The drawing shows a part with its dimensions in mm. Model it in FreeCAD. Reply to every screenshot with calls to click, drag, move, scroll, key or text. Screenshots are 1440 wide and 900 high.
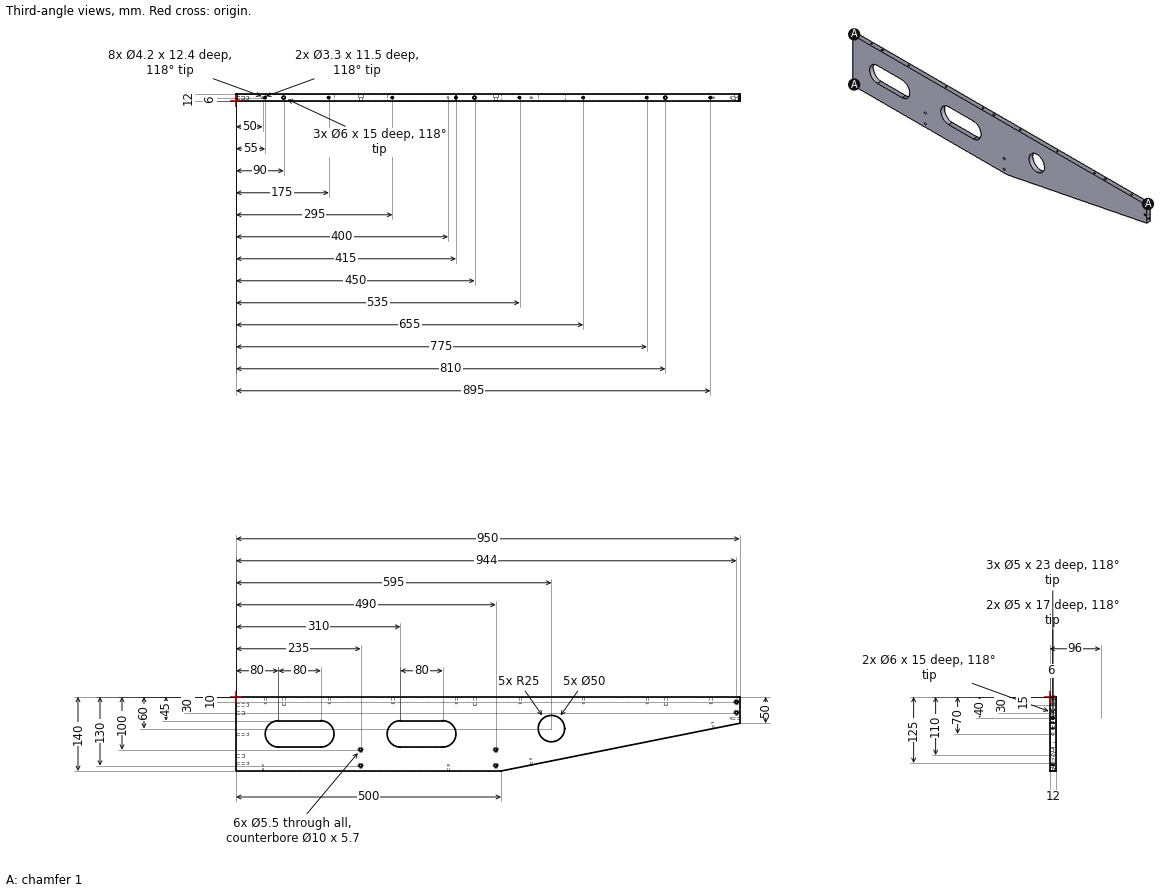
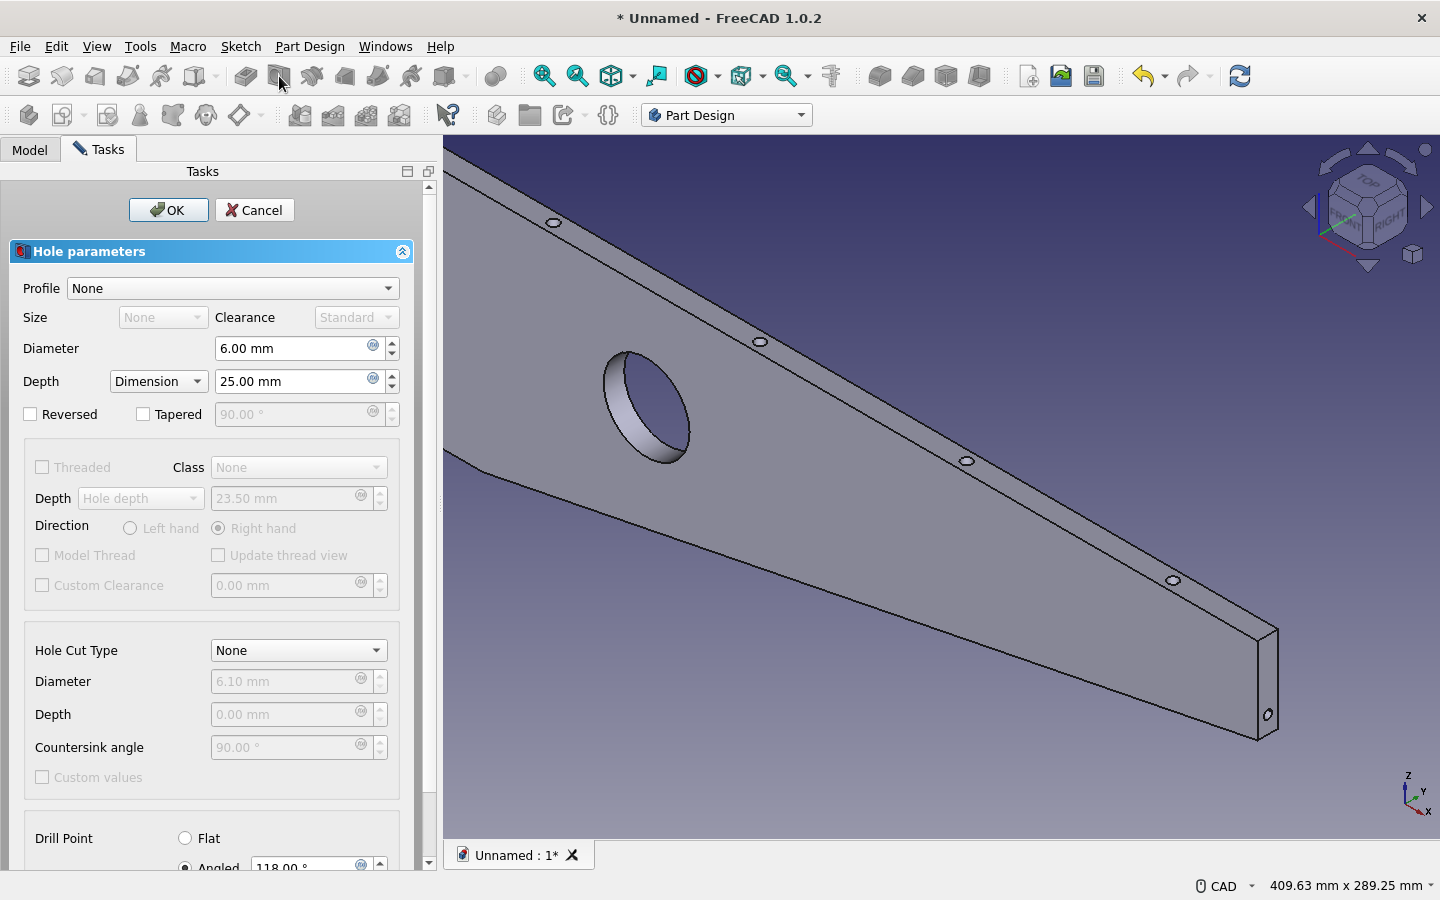
triple_click(300, 348)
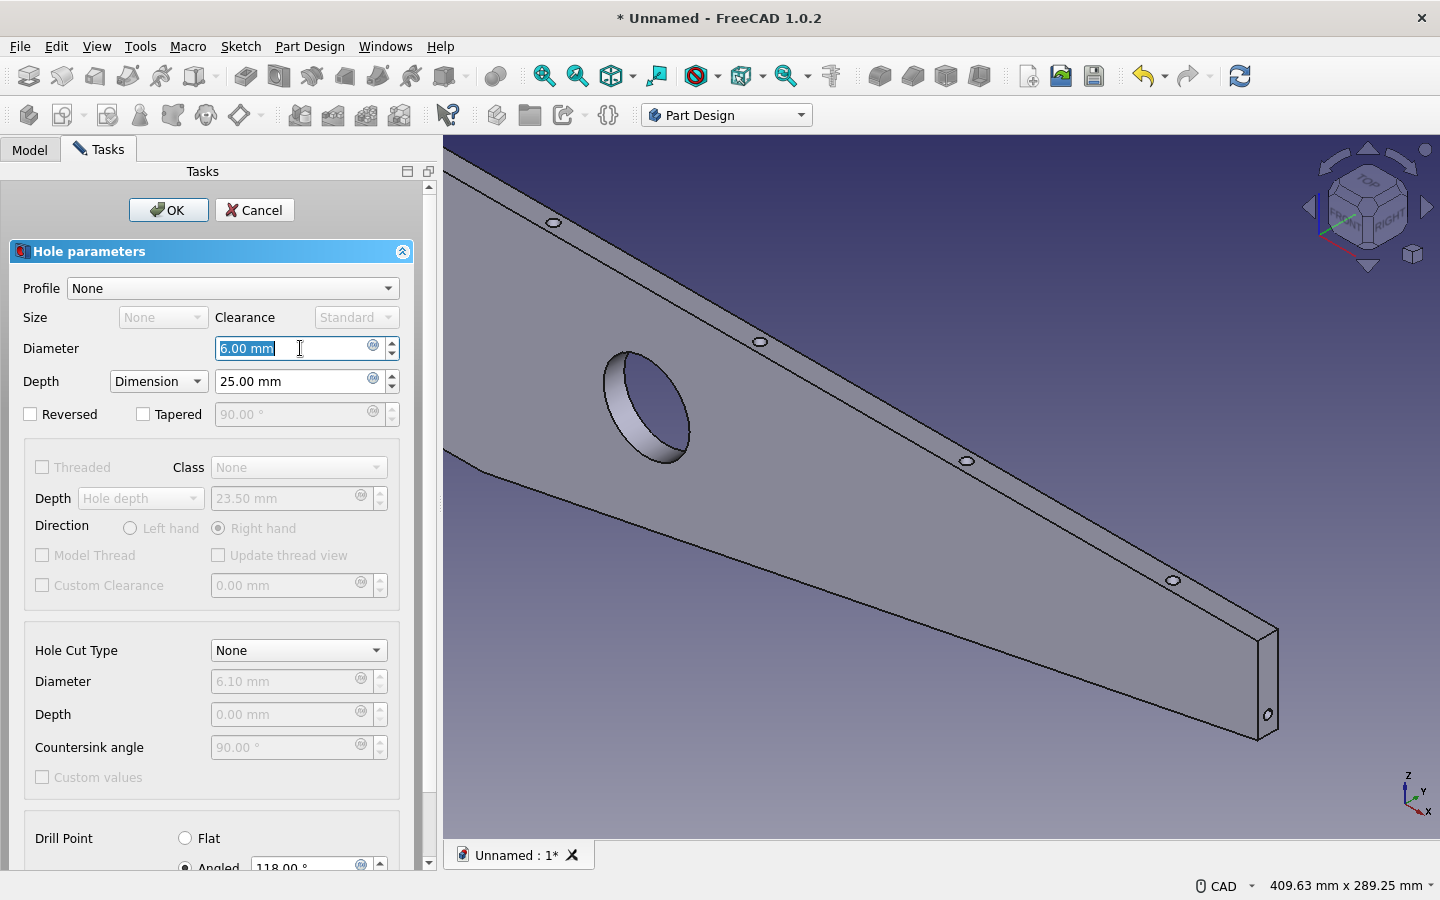
text(4.2)
key(Tab)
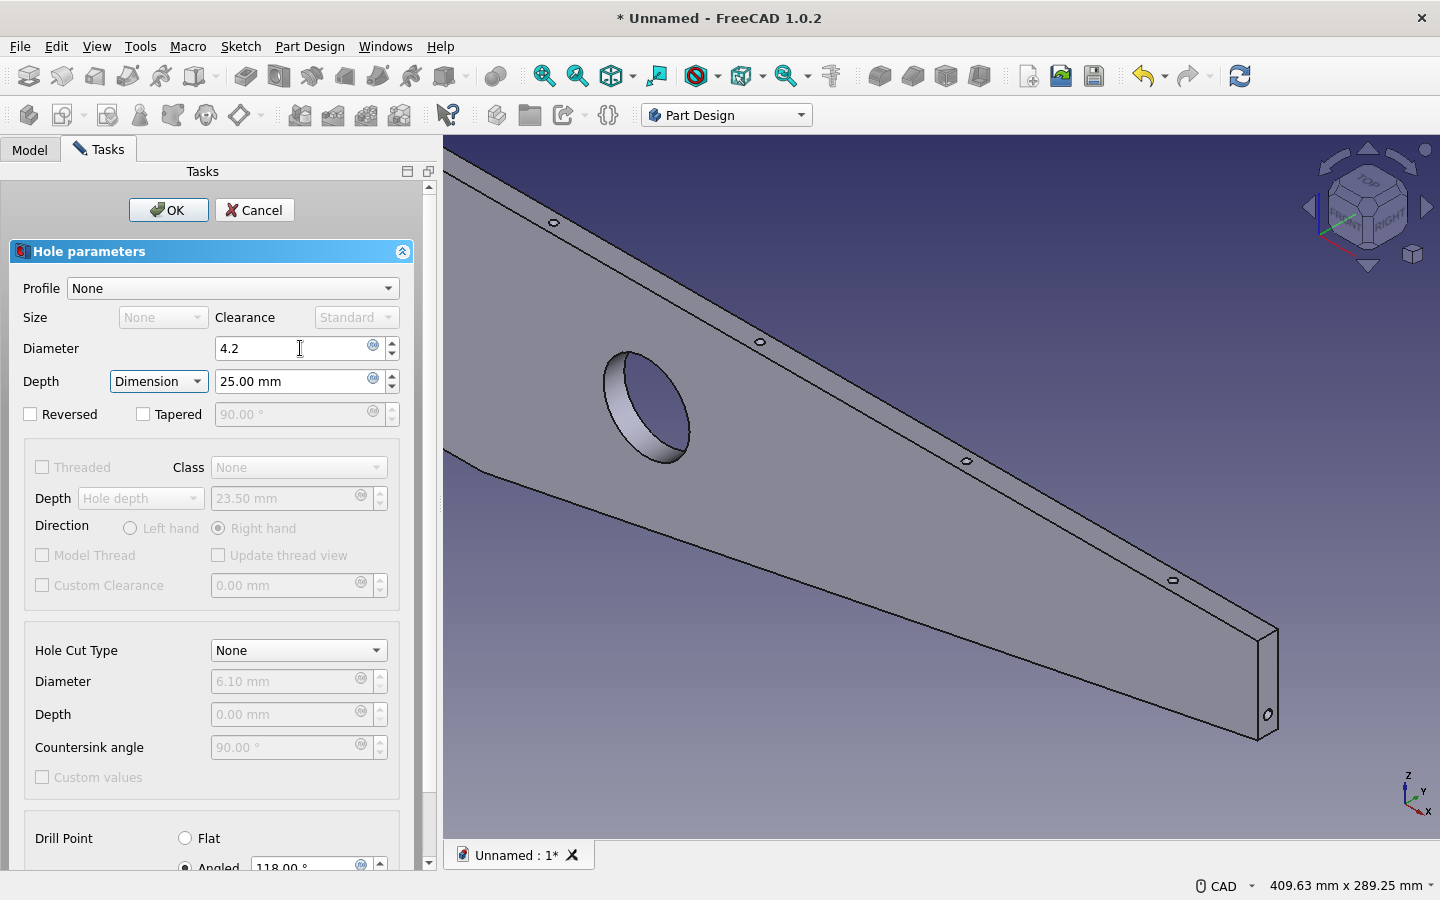
triple_click(300, 382)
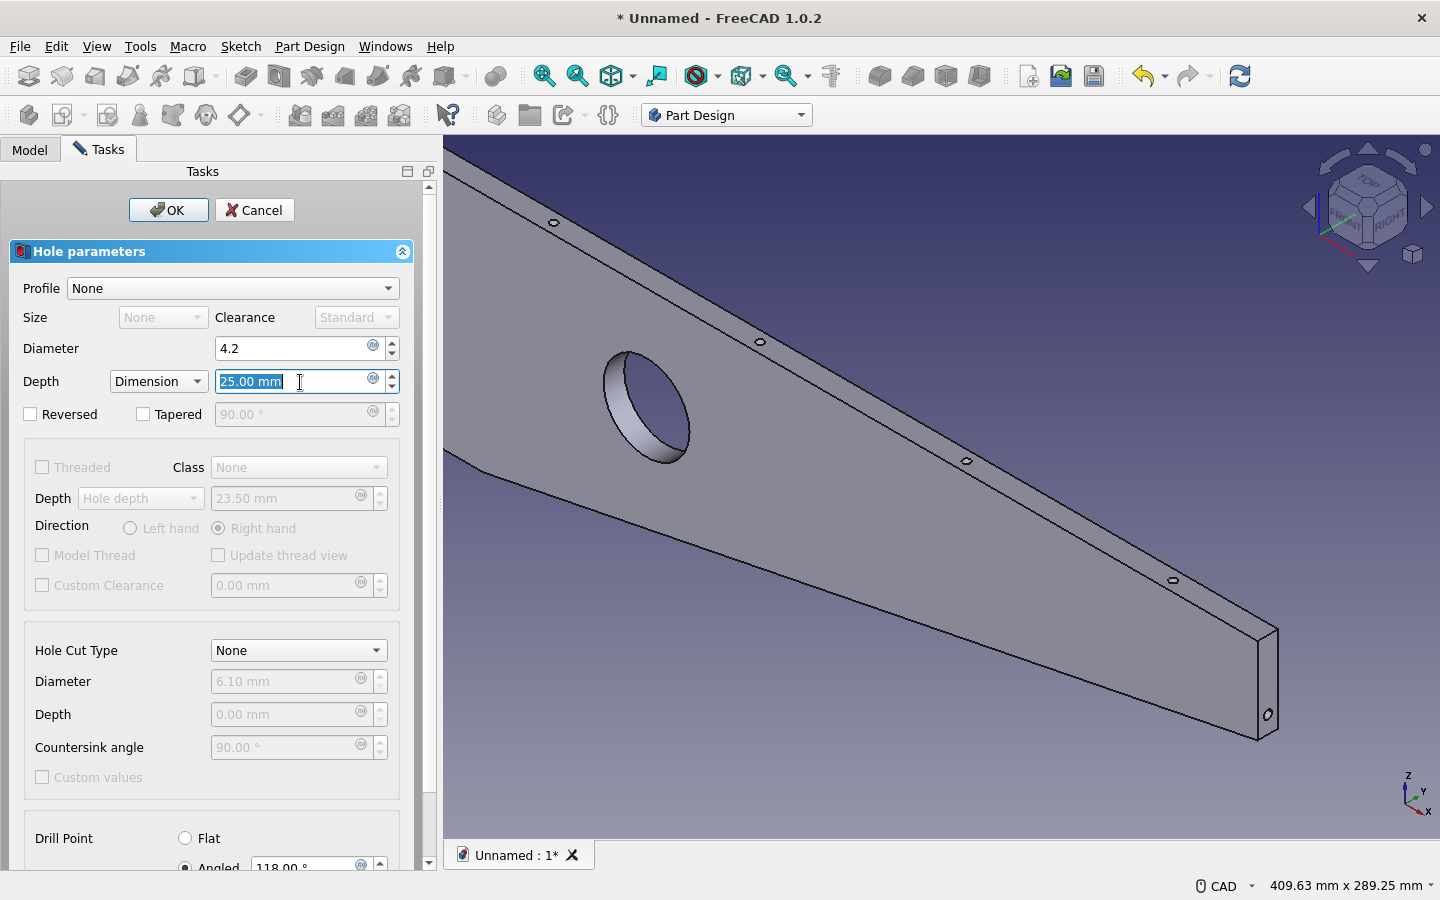
text(12.4)
key(Tab)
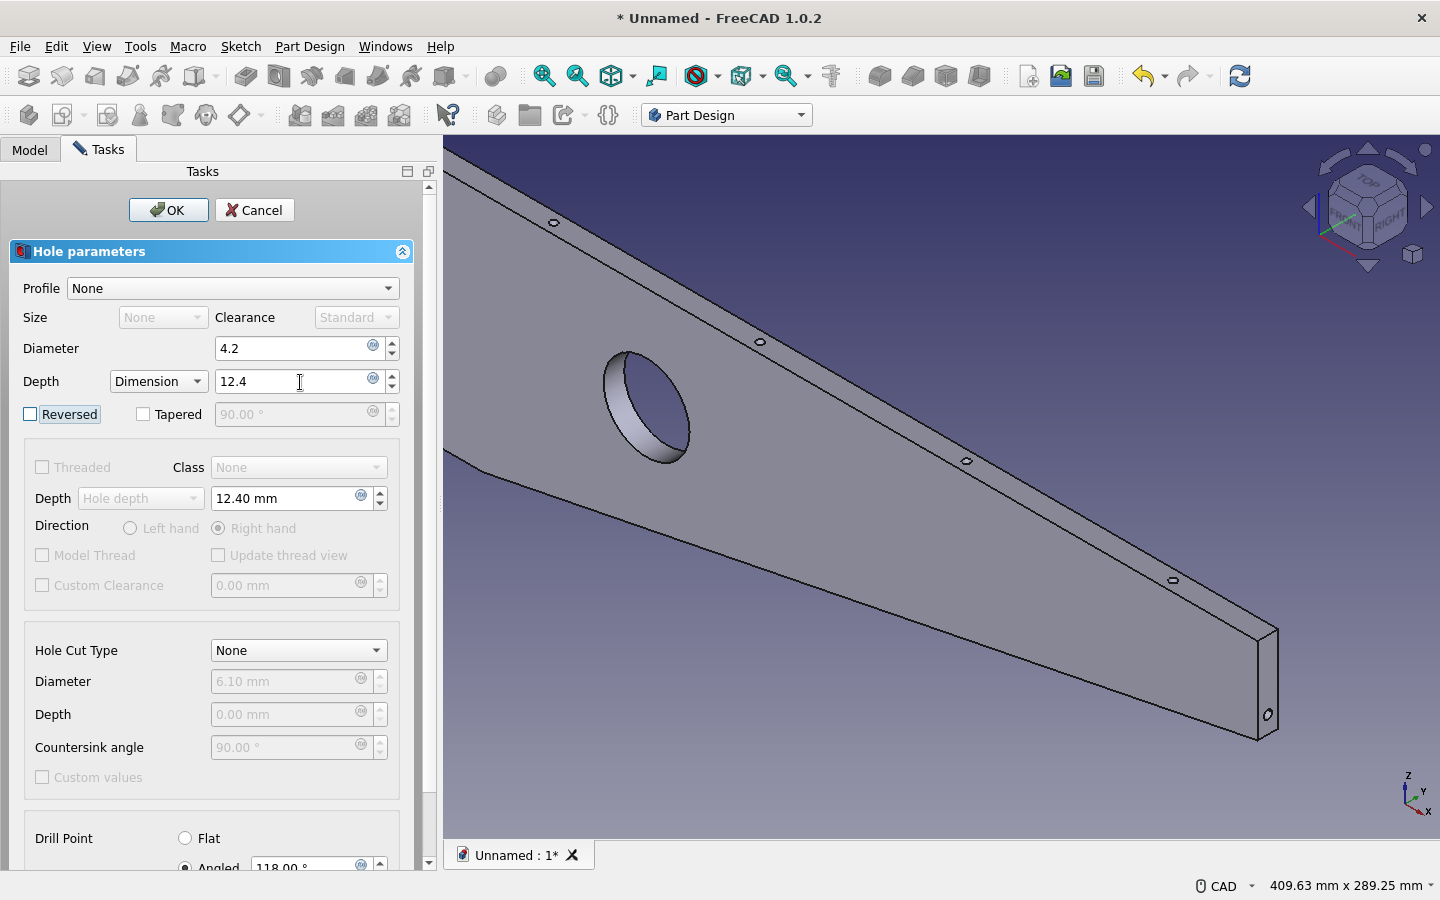
click(169, 210)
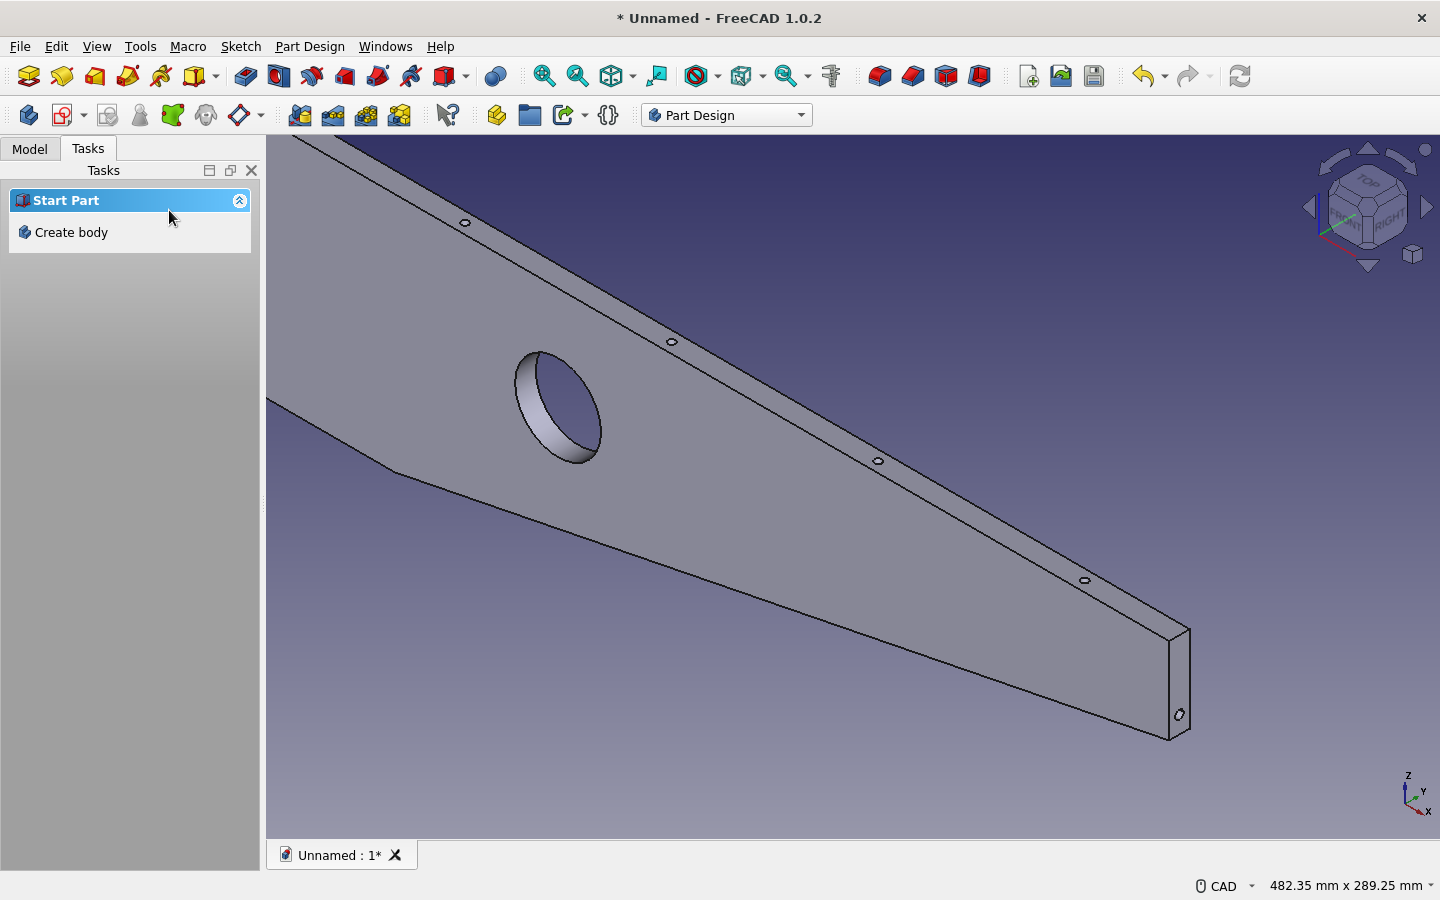
click(545, 76)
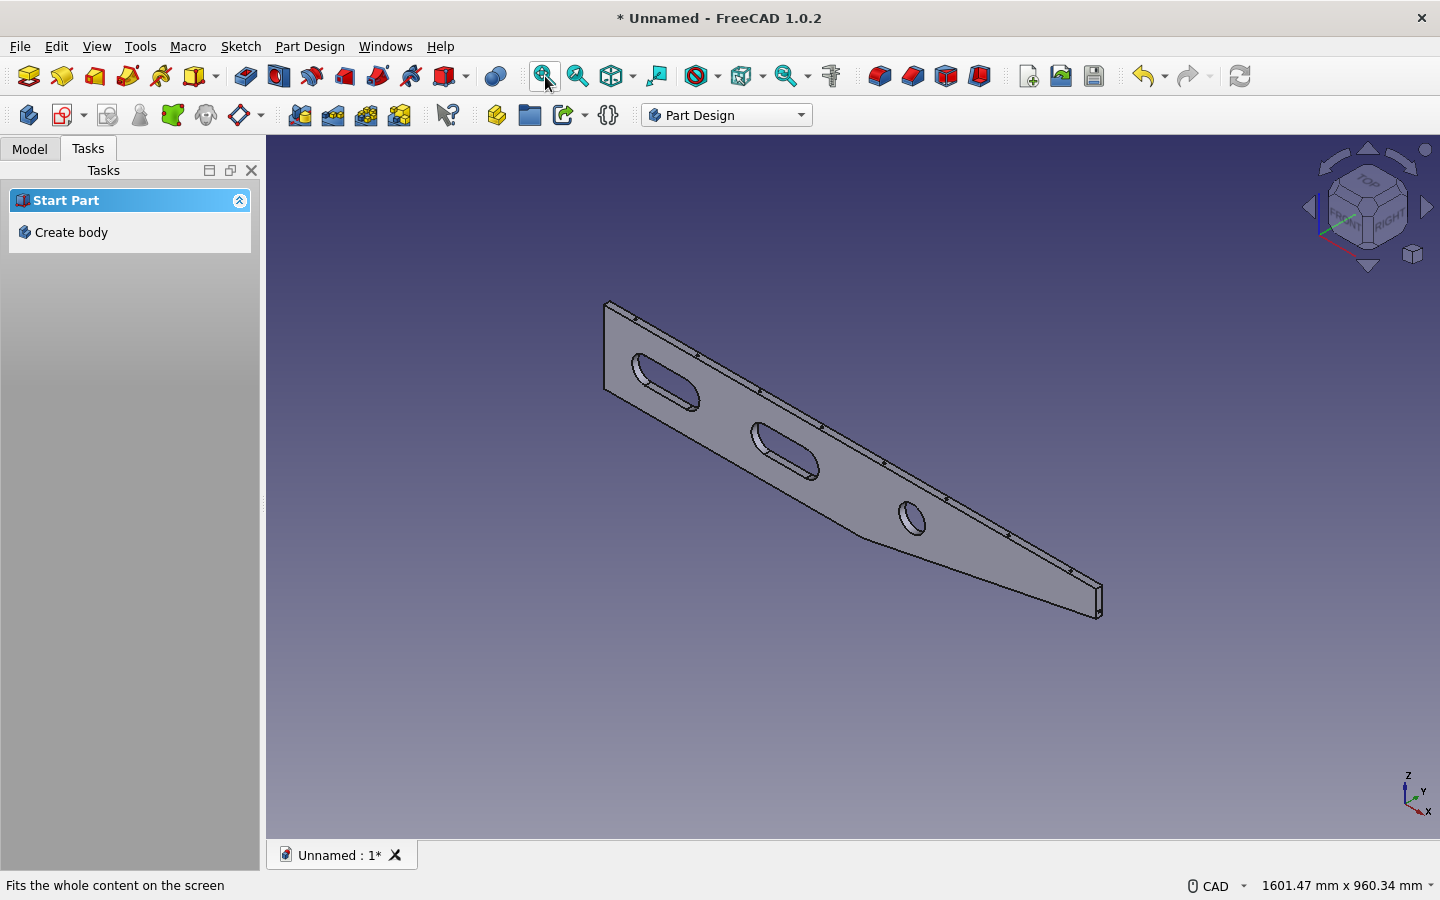
click(62, 116)